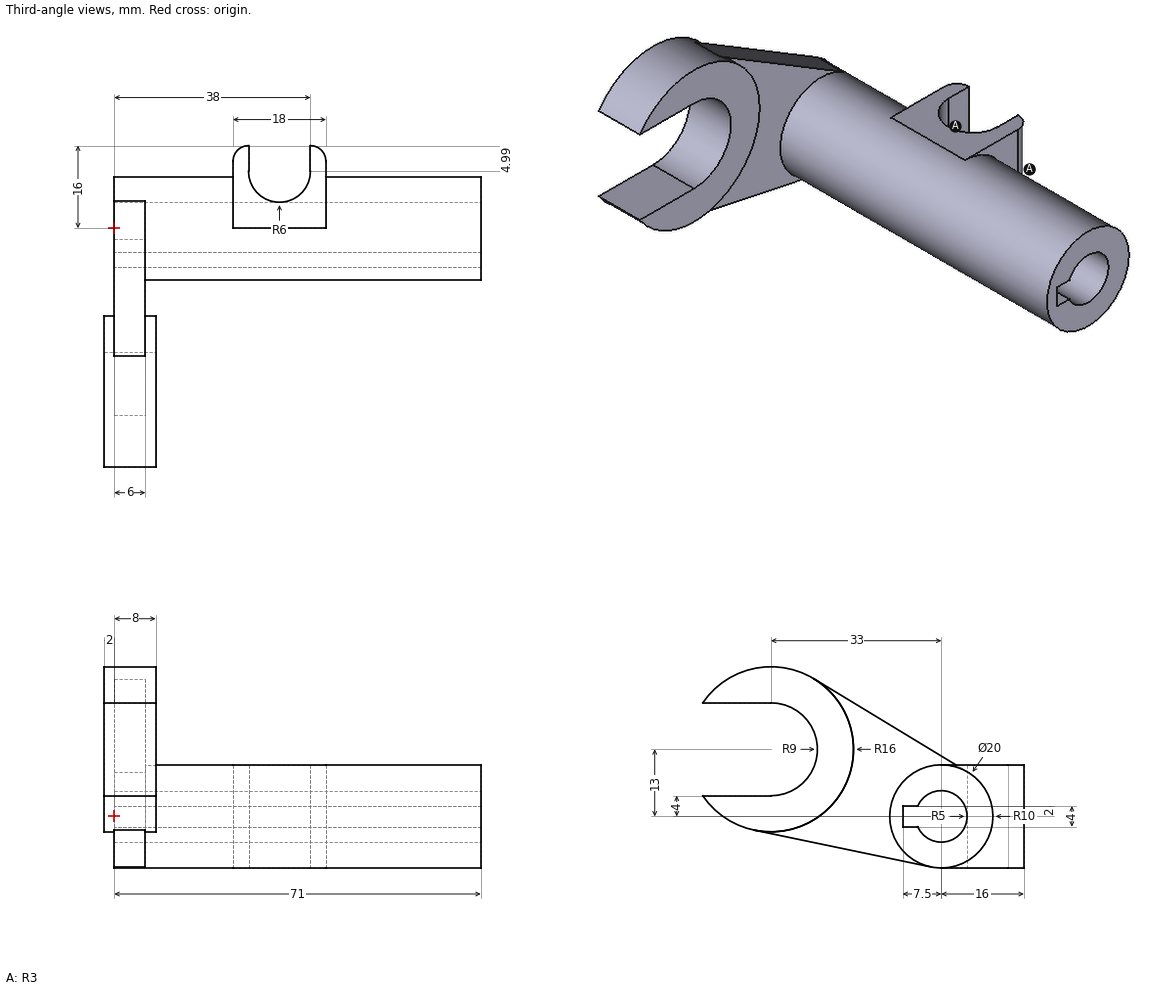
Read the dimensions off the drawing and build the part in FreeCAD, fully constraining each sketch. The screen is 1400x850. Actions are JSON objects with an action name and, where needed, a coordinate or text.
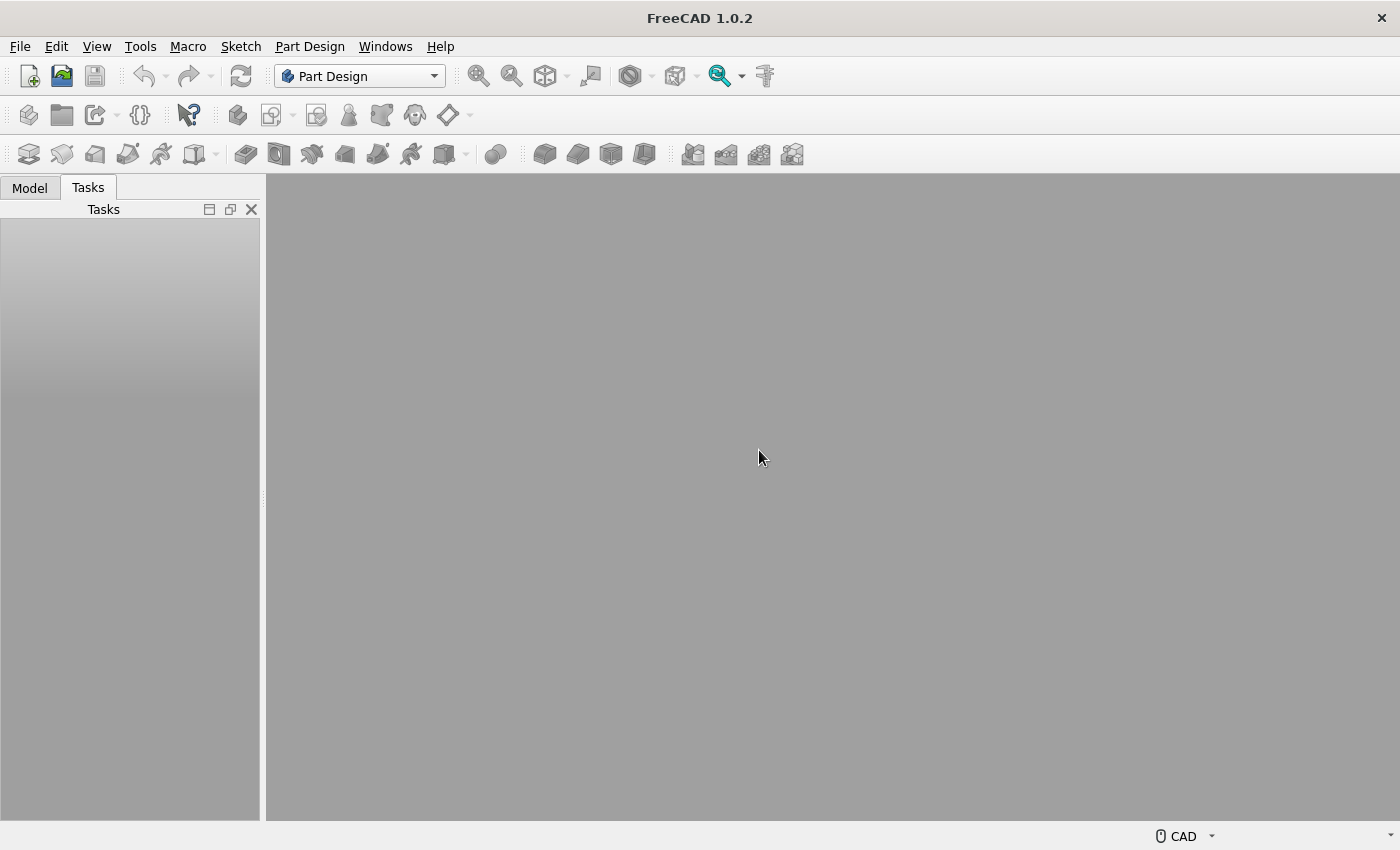
{"action": "key", "text": "ctrl+n"}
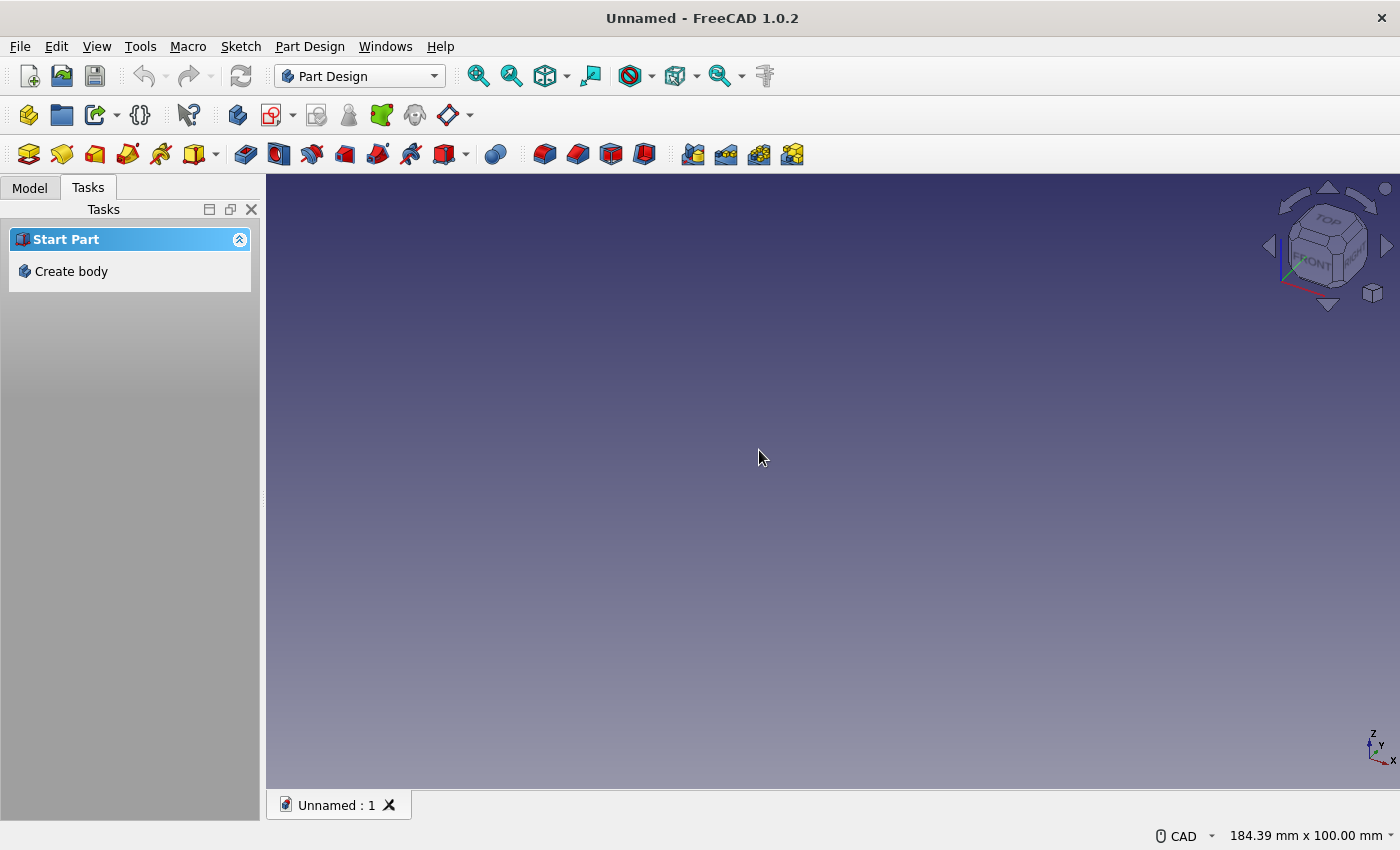
{"action": "left_click", "coordinate": [270, 116]}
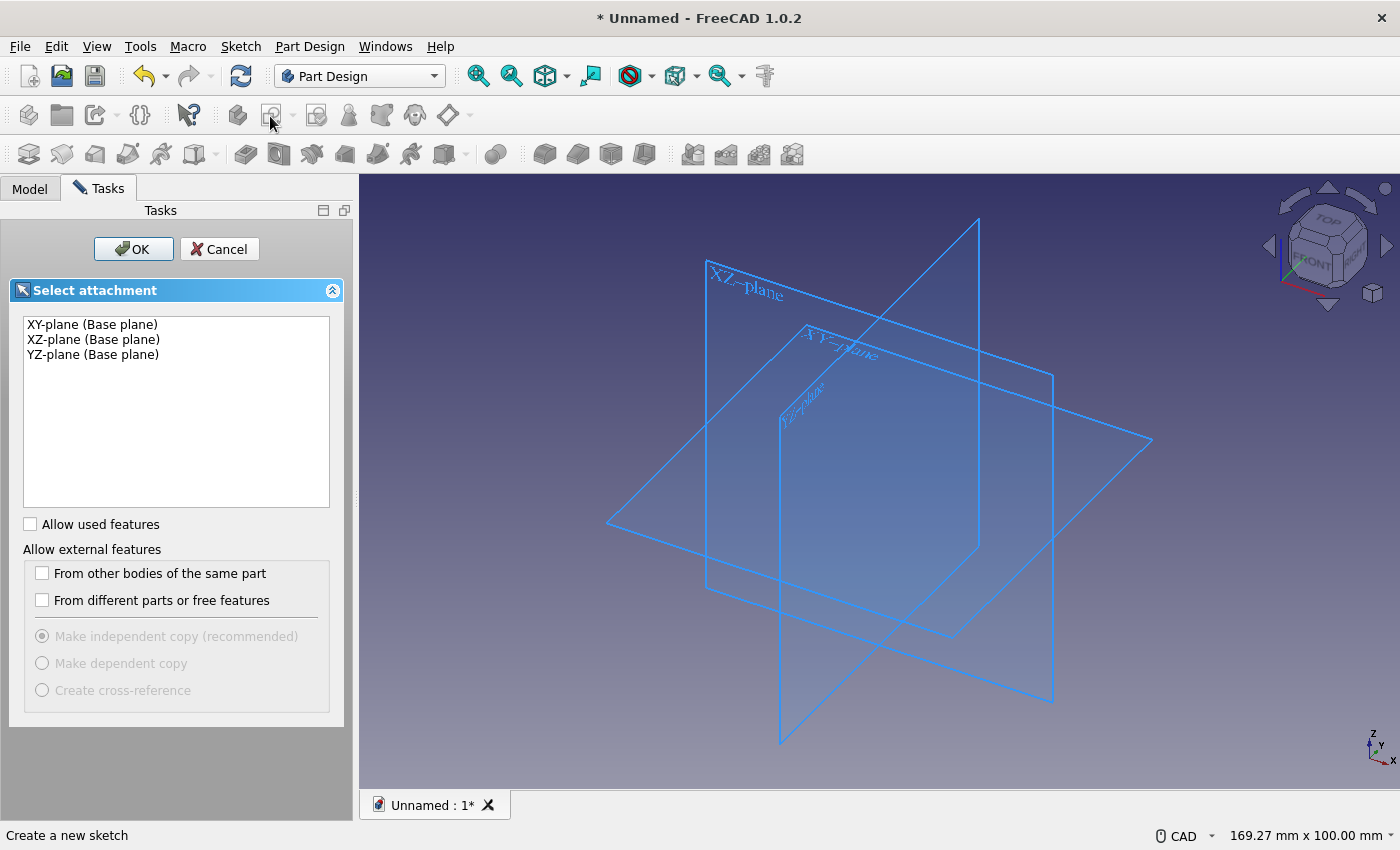
{"action": "left_click", "coordinate": [84, 354]}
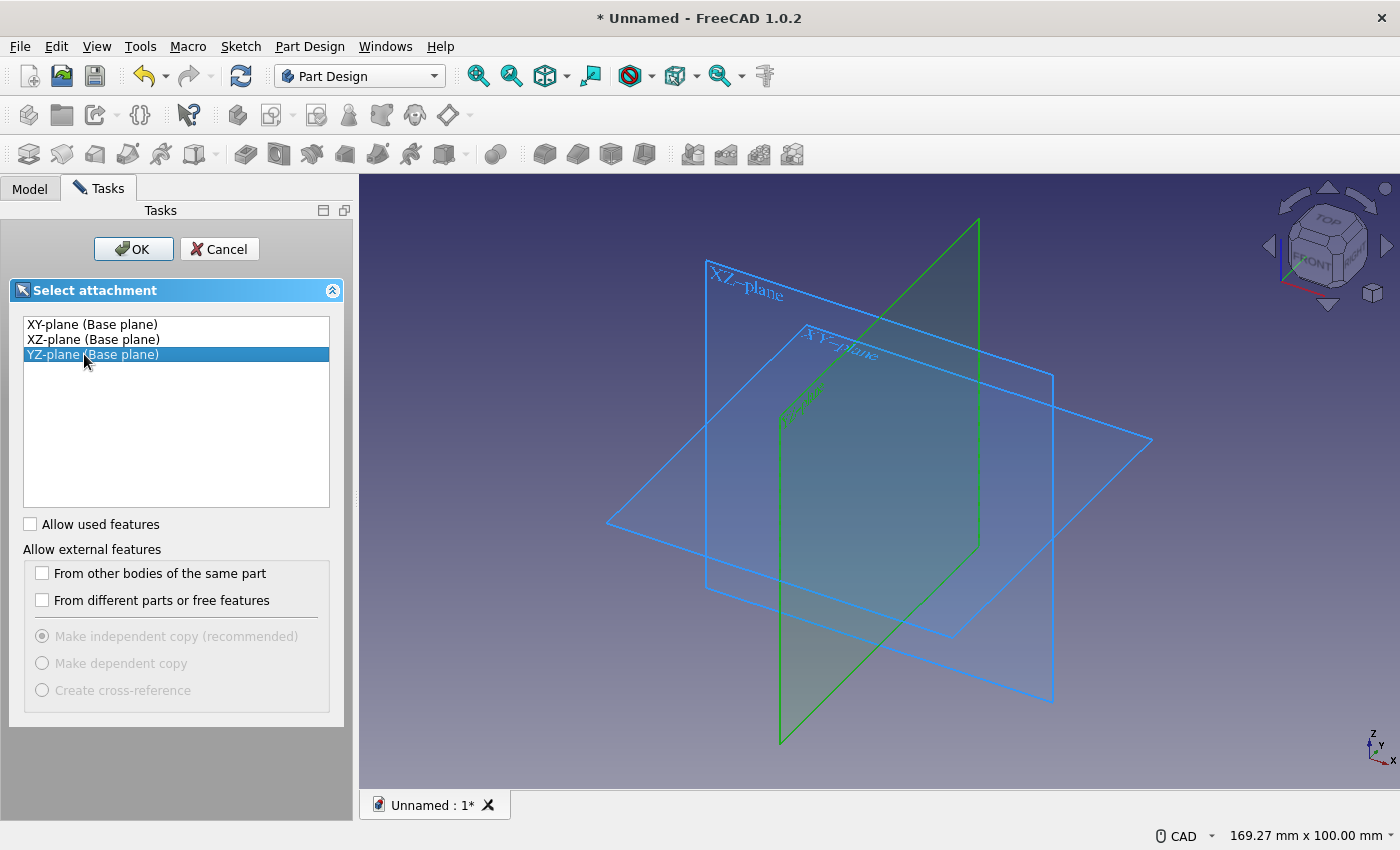
{"action": "left_click", "coordinate": [134, 249]}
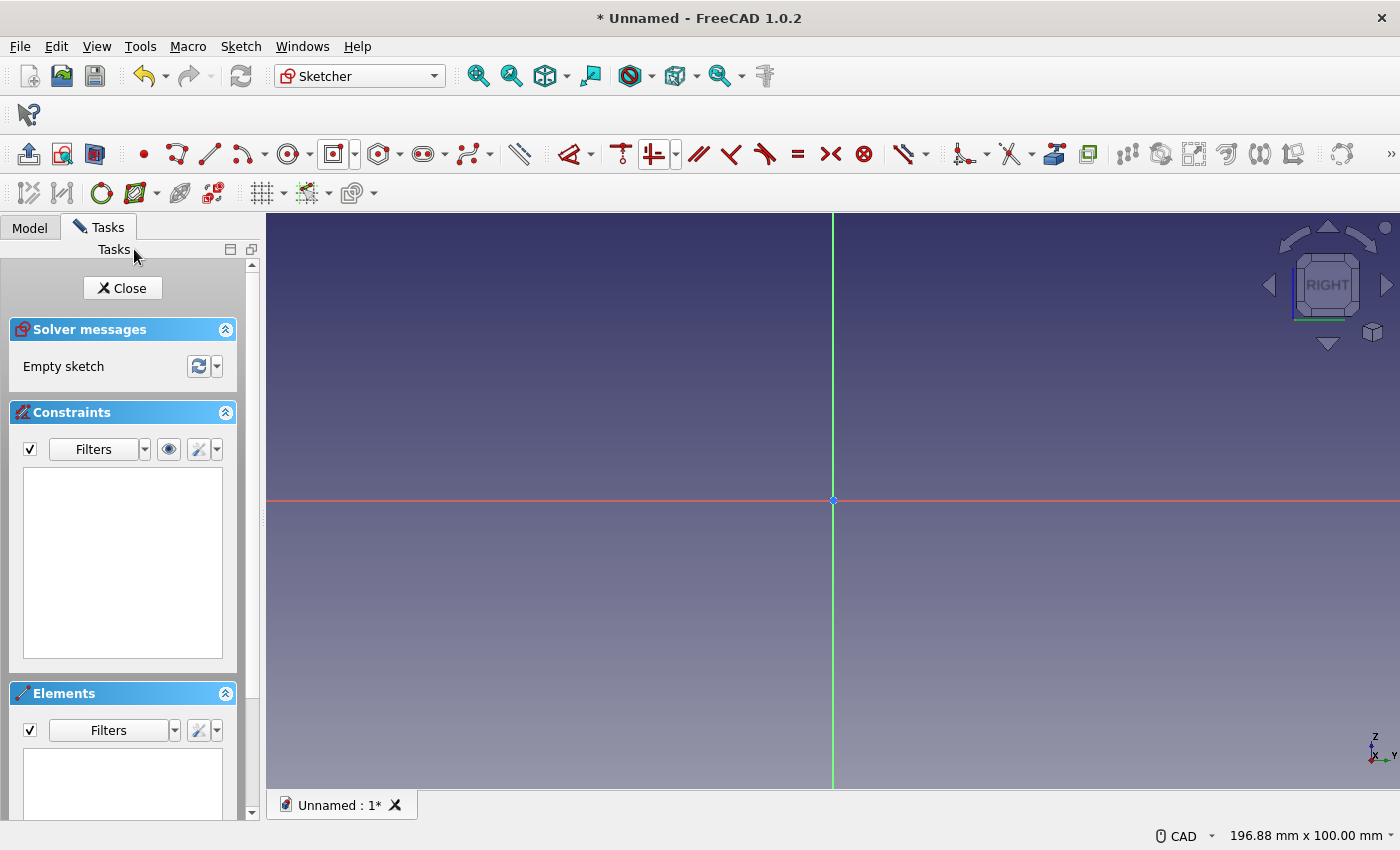
{"action": "scroll", "coordinate": [863, 501], "scroll_direction": "up", "scroll_amount": 6}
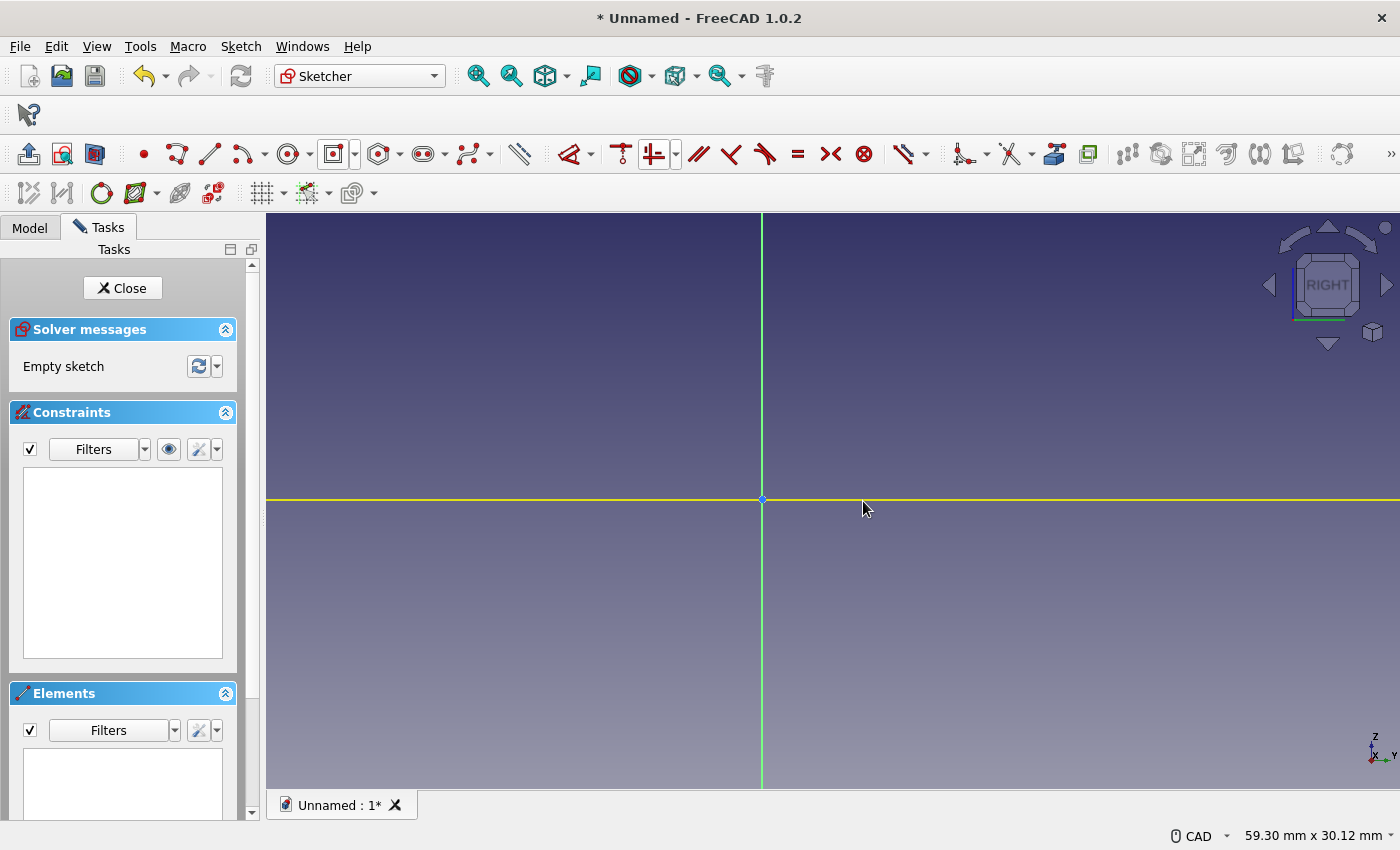
{"action": "key", "text": "g c"}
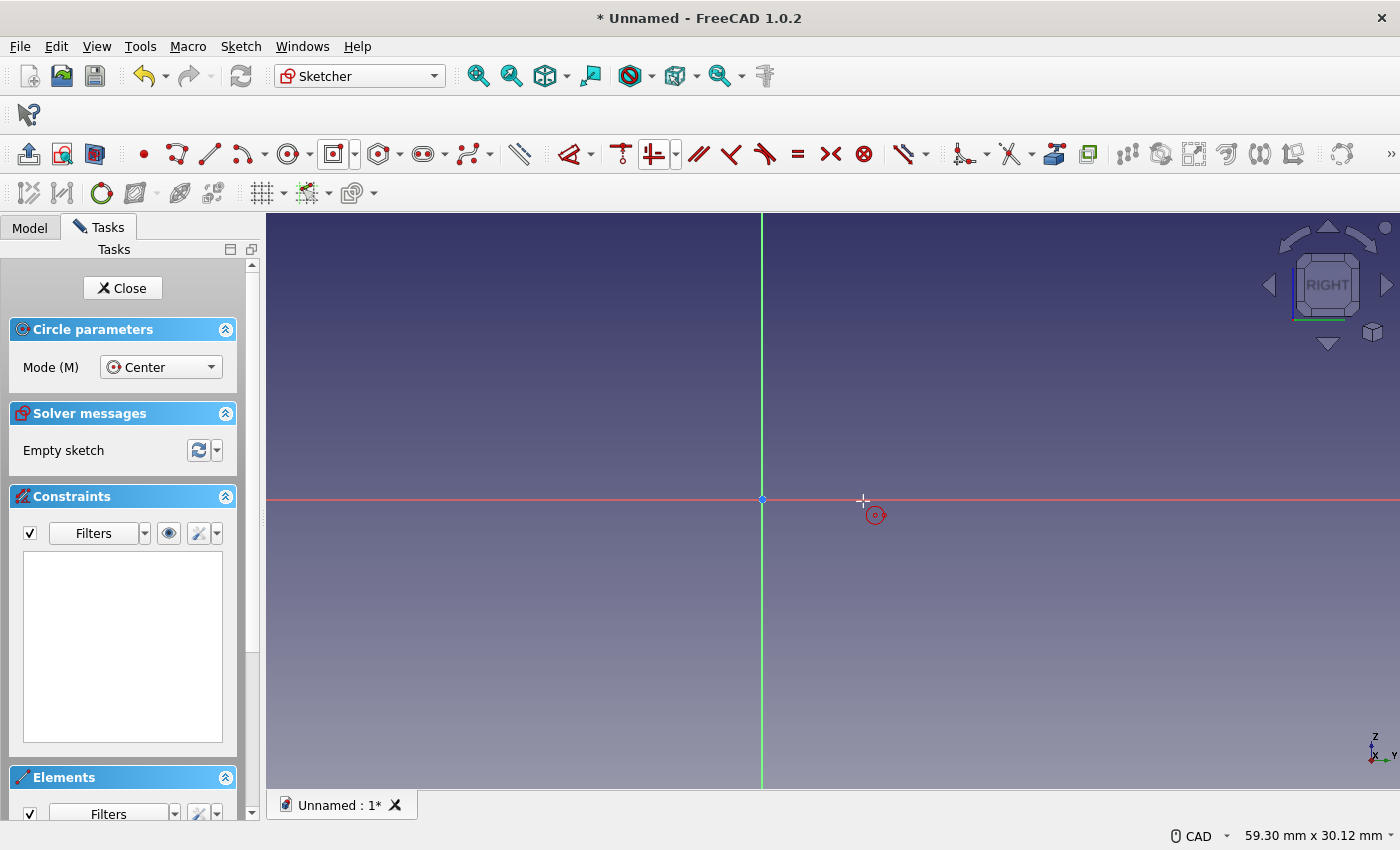
{"action": "left_click", "coordinate": [762, 500]}
{"action": "left_click", "coordinate": [897, 365]}
{"action": "key", "text": "Escape"}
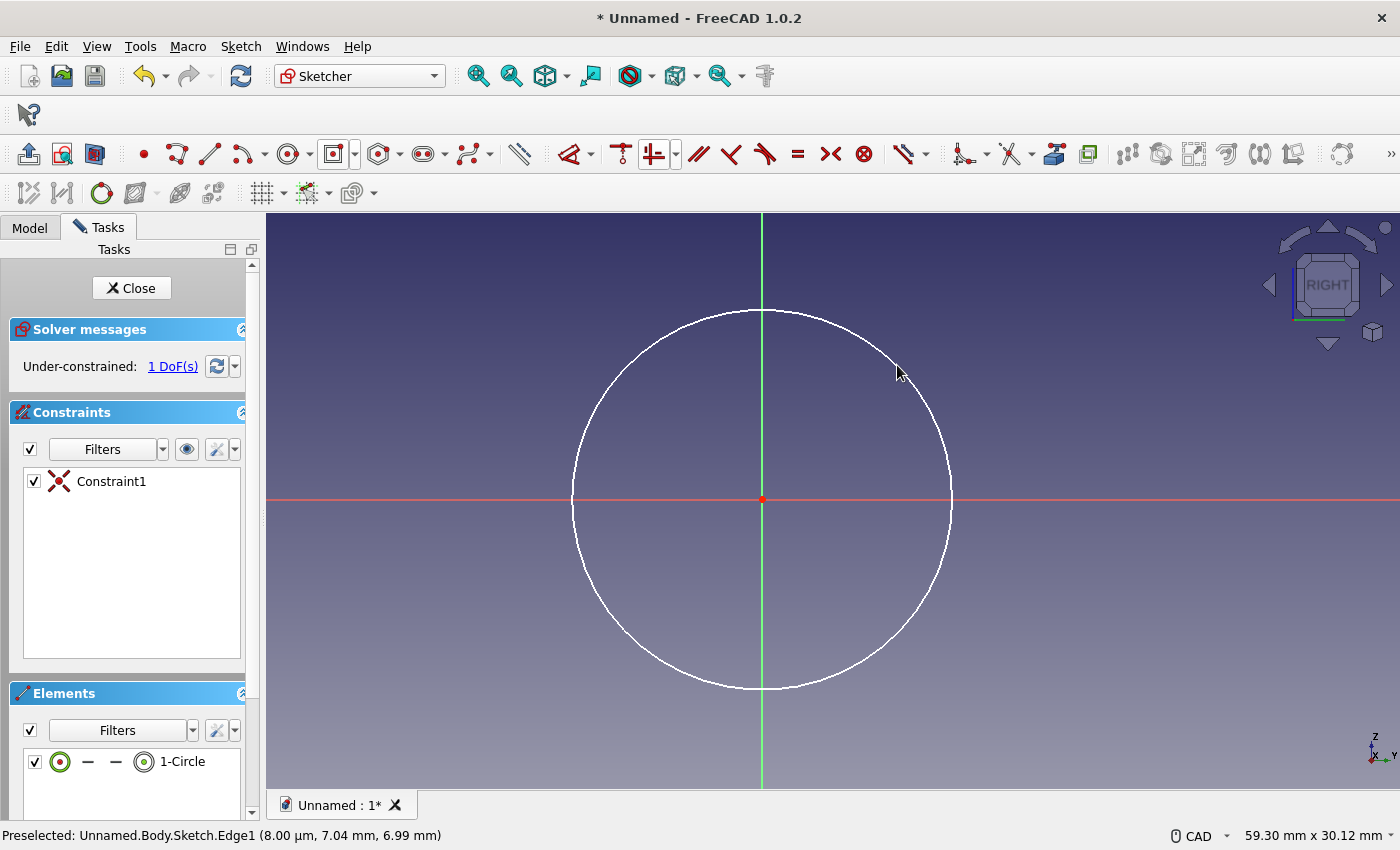
{"action": "key", "text": "d"}